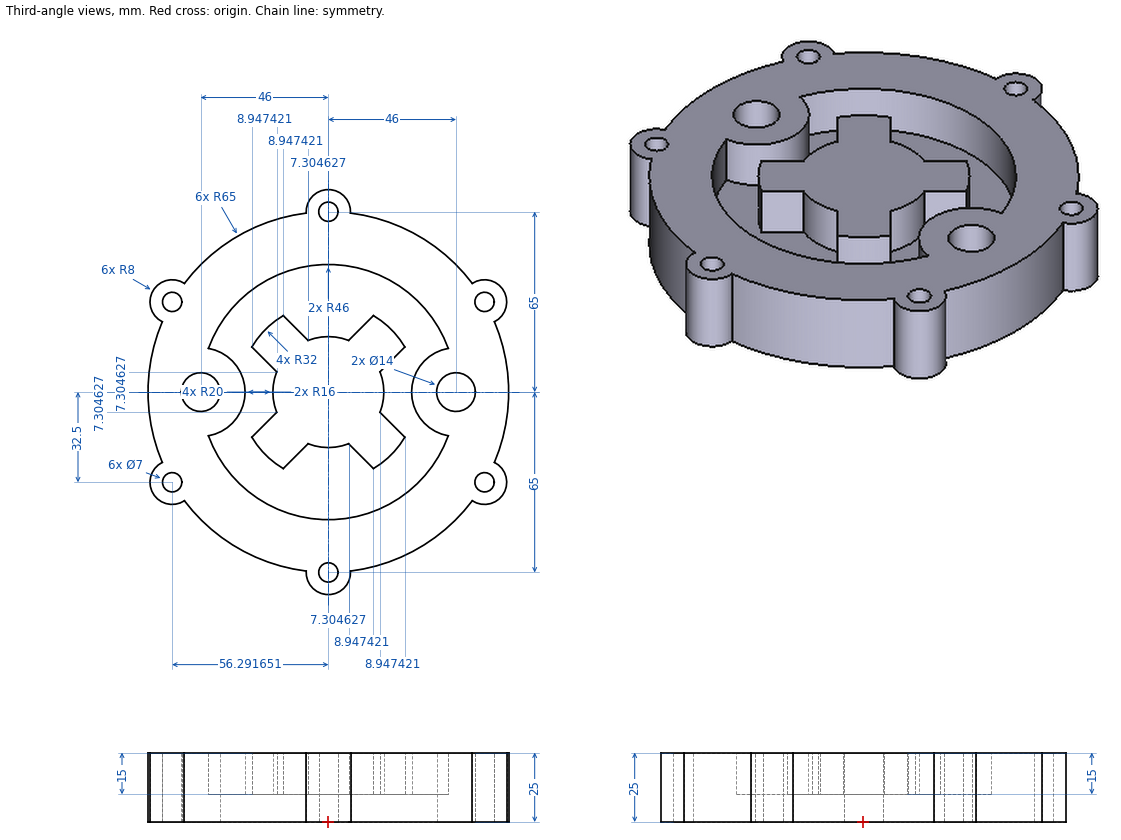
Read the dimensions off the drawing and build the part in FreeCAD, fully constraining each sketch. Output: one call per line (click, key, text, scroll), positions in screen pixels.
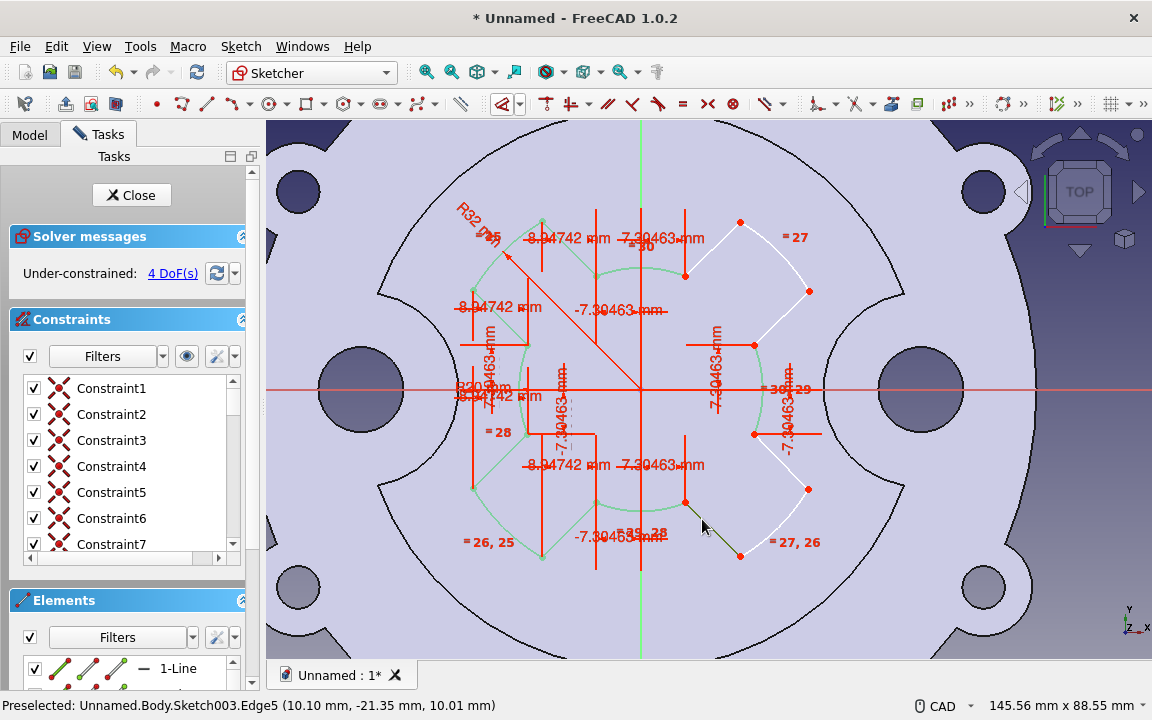
click(520, 104)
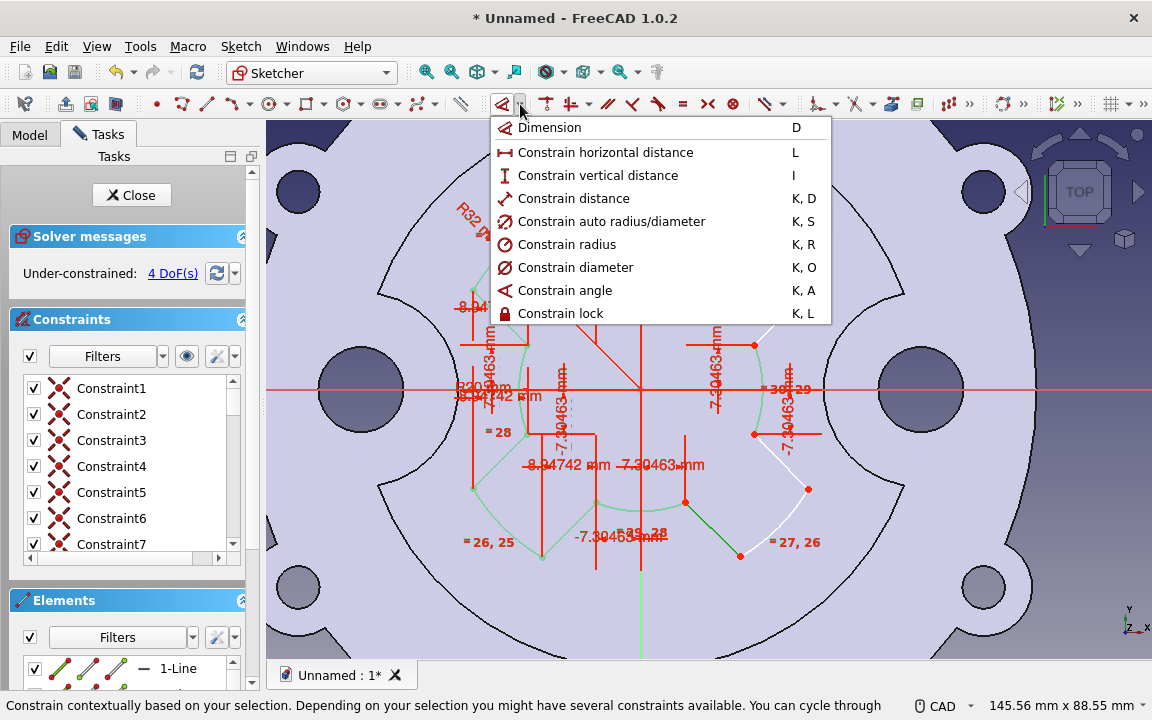
click(661, 152)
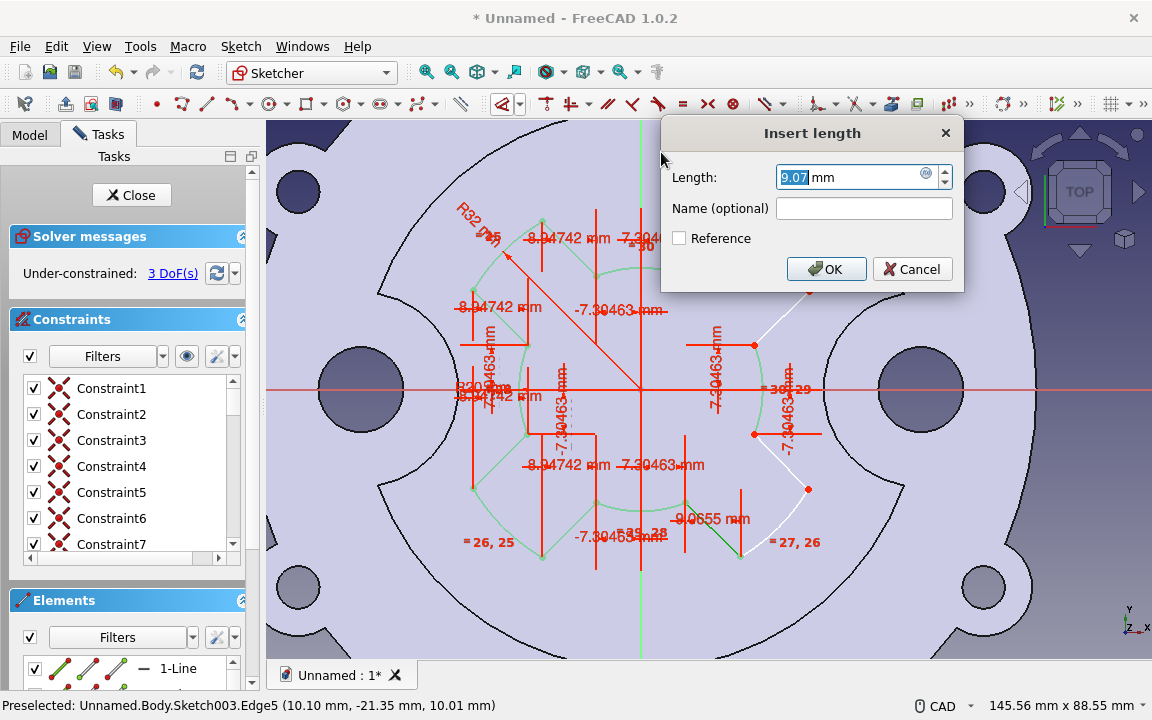
text(8.947421)
key(Return)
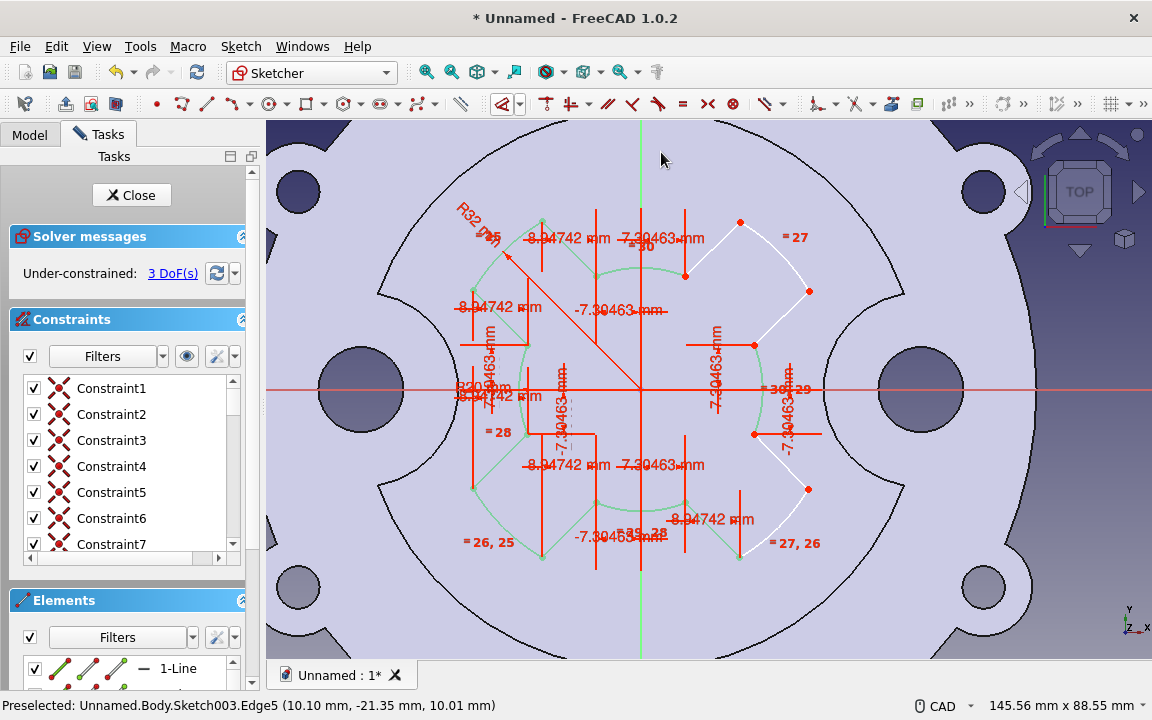
click(792, 473)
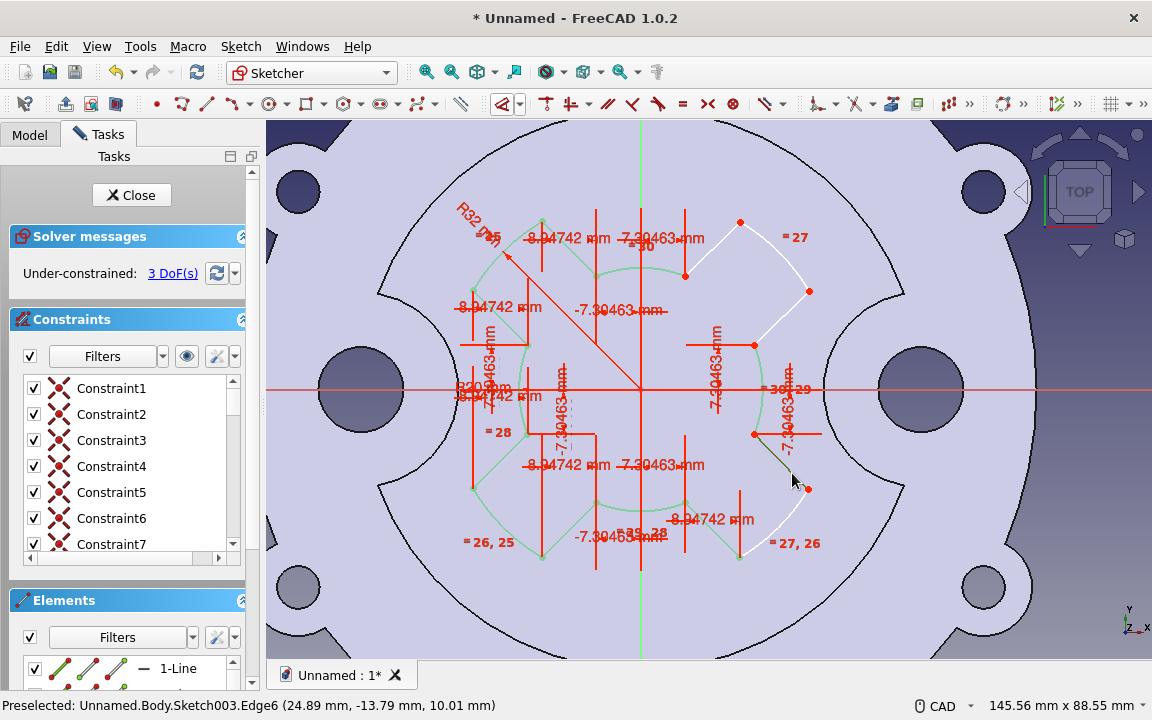
key(l)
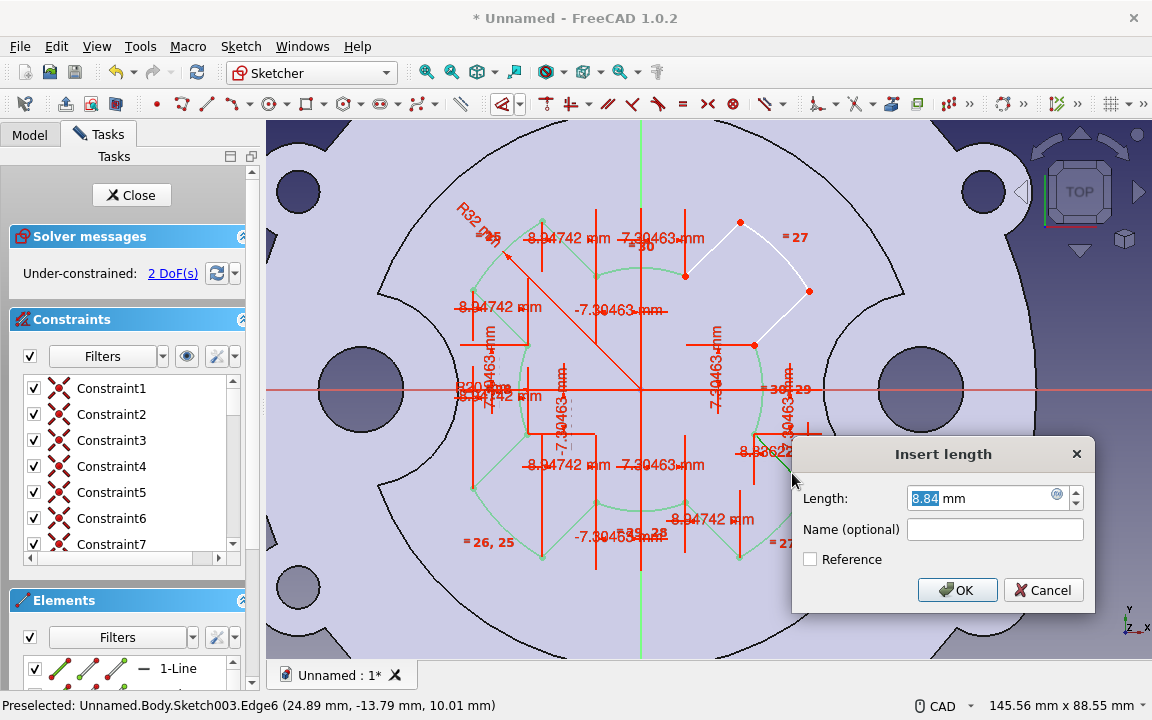
text(8.947421)
key(Return)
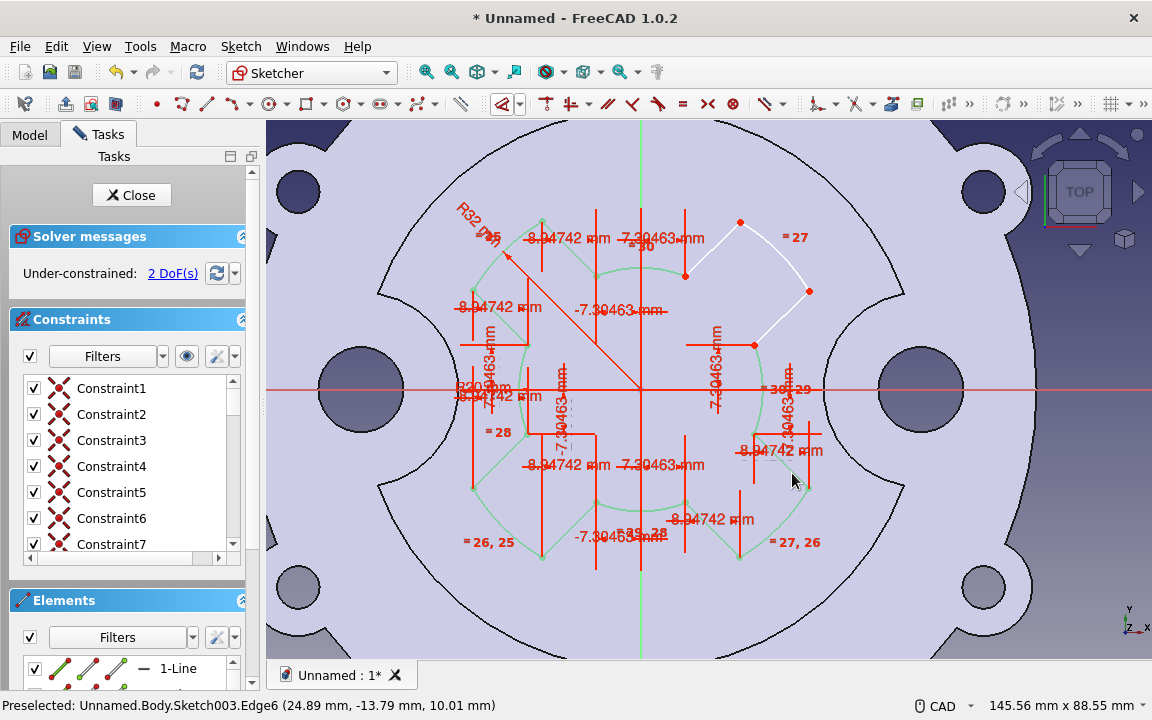
click(771, 329)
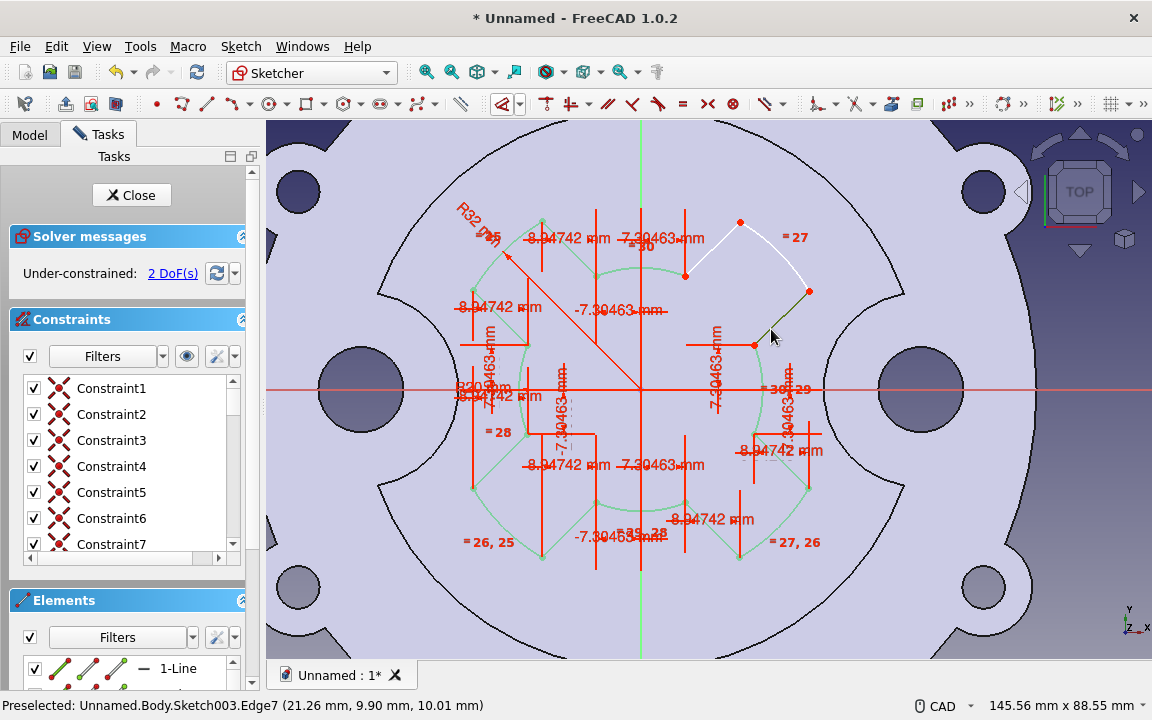
click(520, 104)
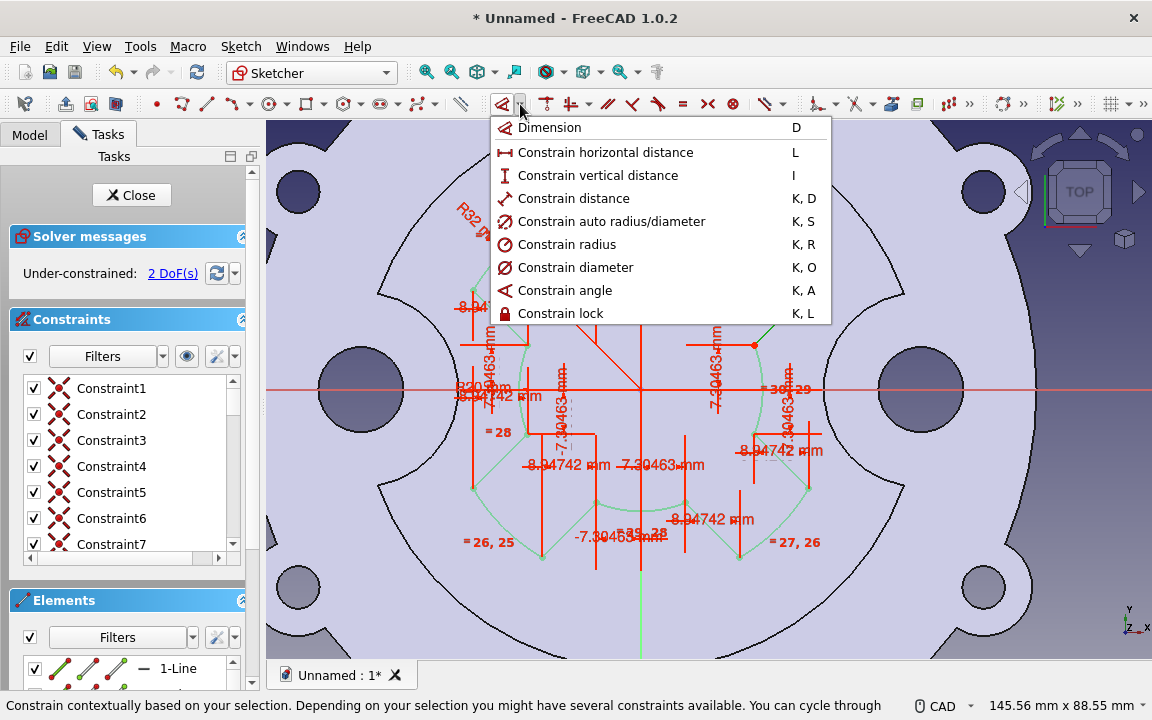
click(661, 152)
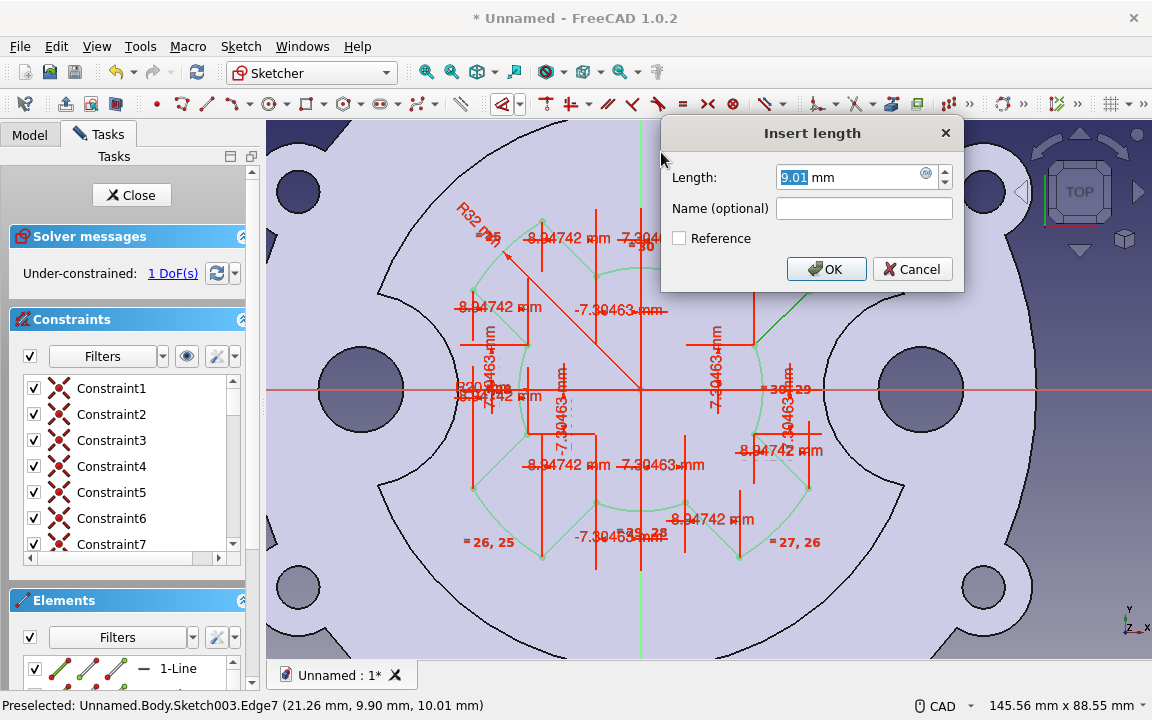
text(8.947421)
key(Return)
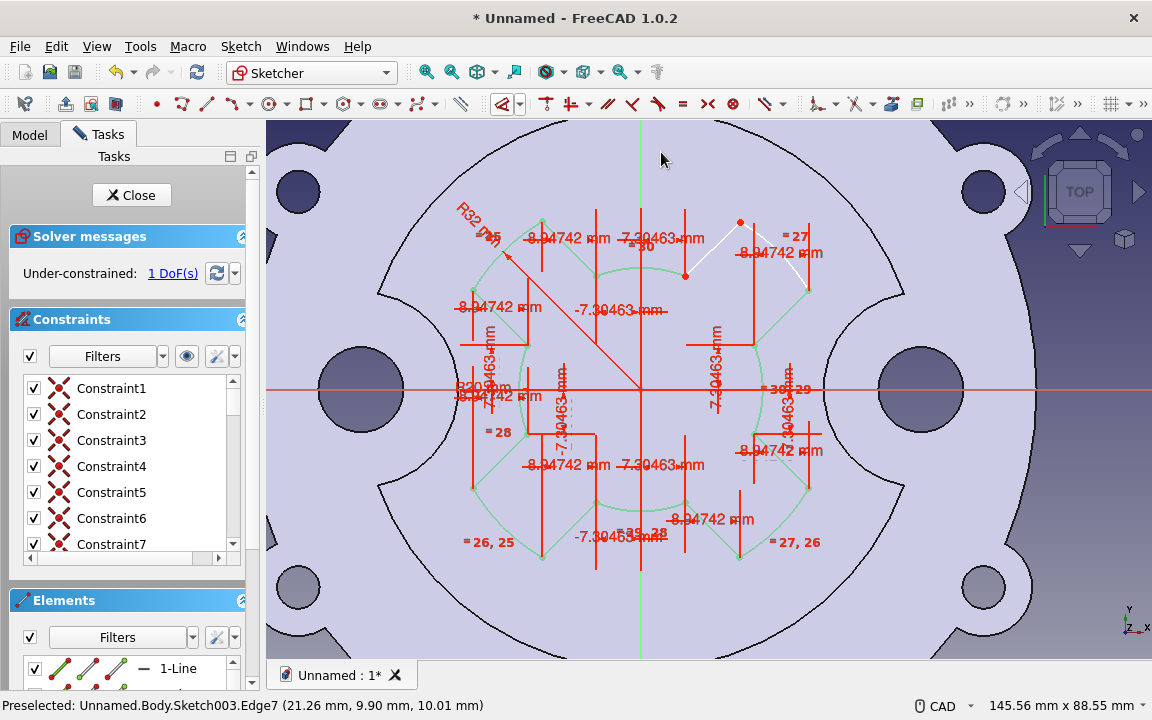
click(724, 238)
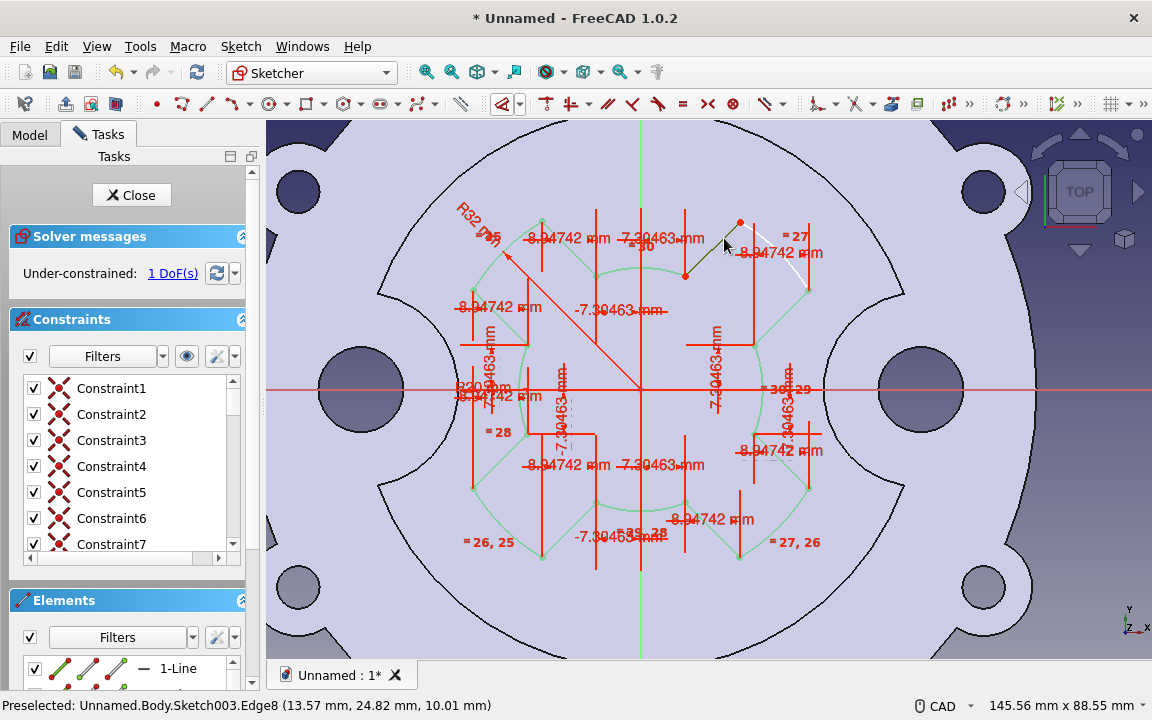
key(l)